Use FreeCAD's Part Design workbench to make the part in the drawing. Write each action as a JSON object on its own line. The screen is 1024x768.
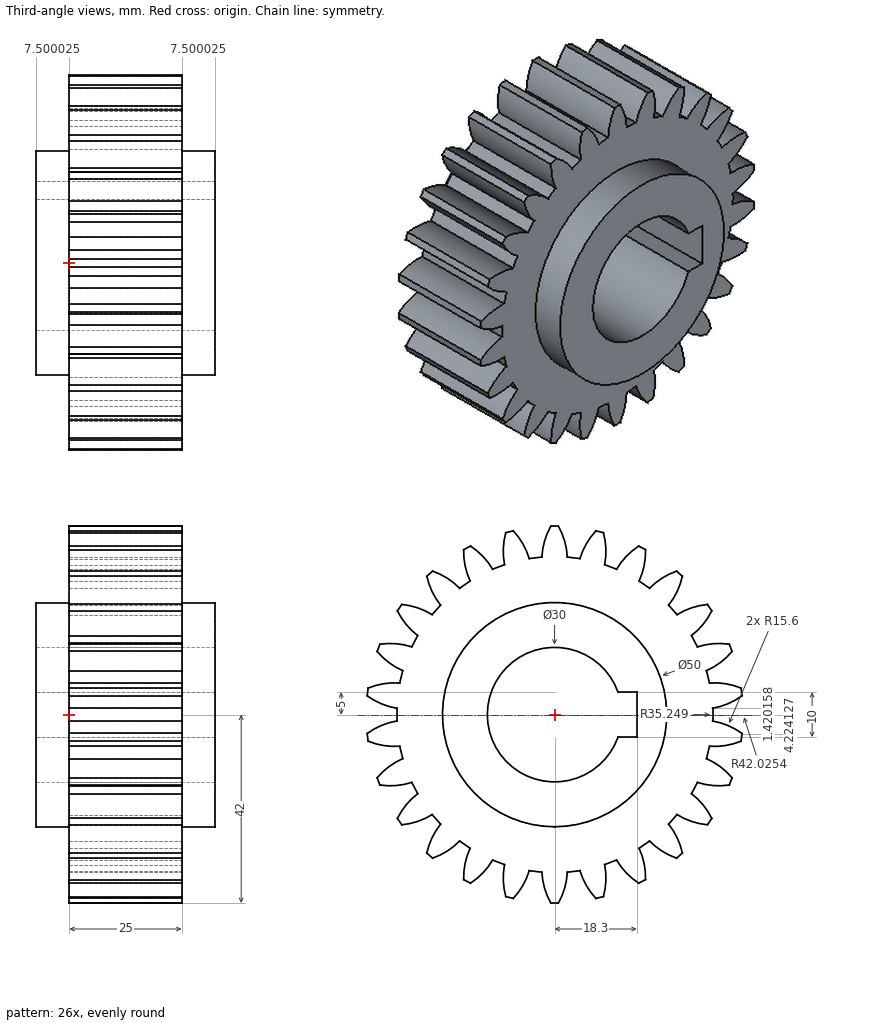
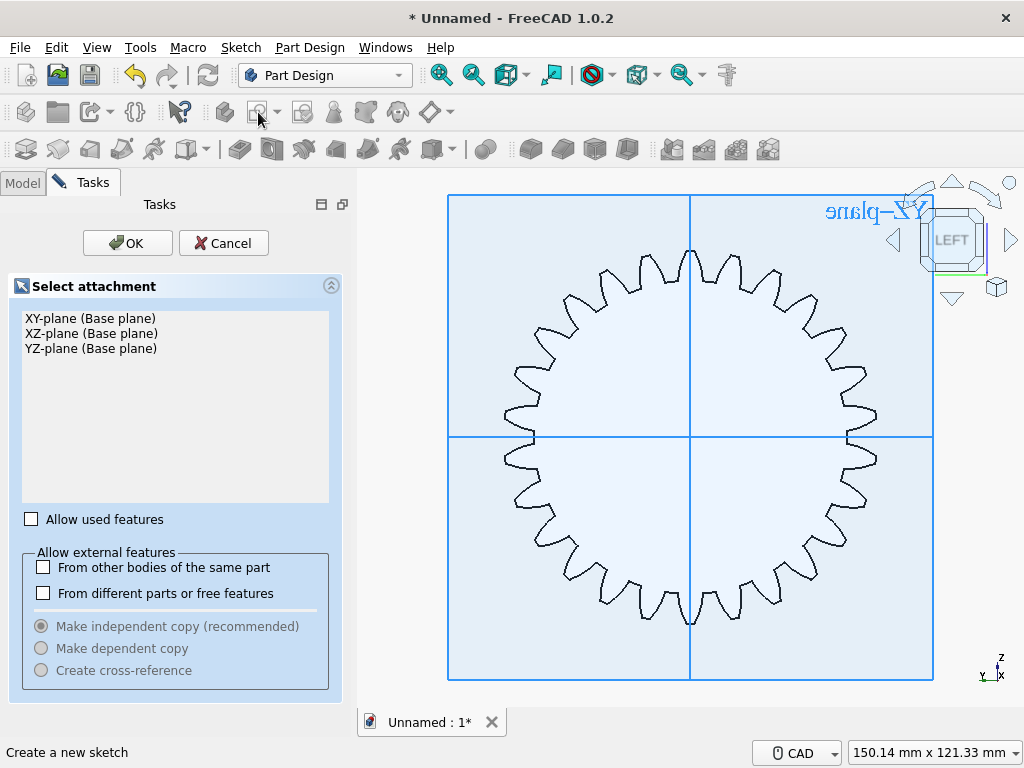
{"action": "left_click", "coordinate": [82, 348]}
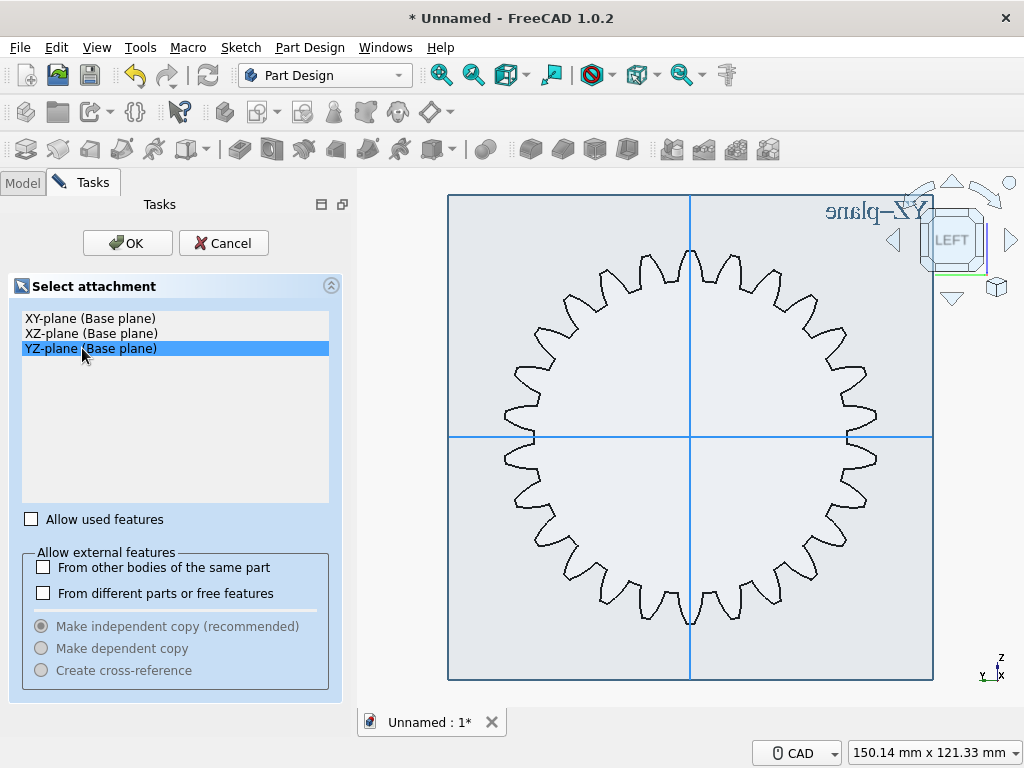
{"action": "left_click", "coordinate": [128, 243]}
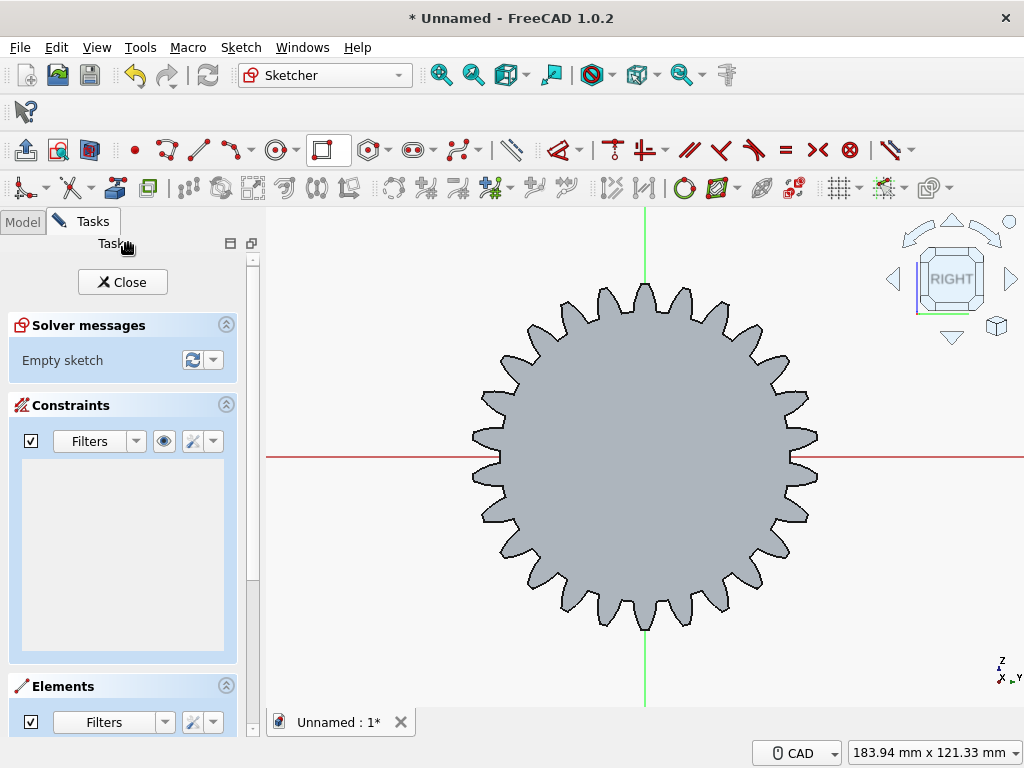
{"action": "left_click", "coordinate": [90, 150]}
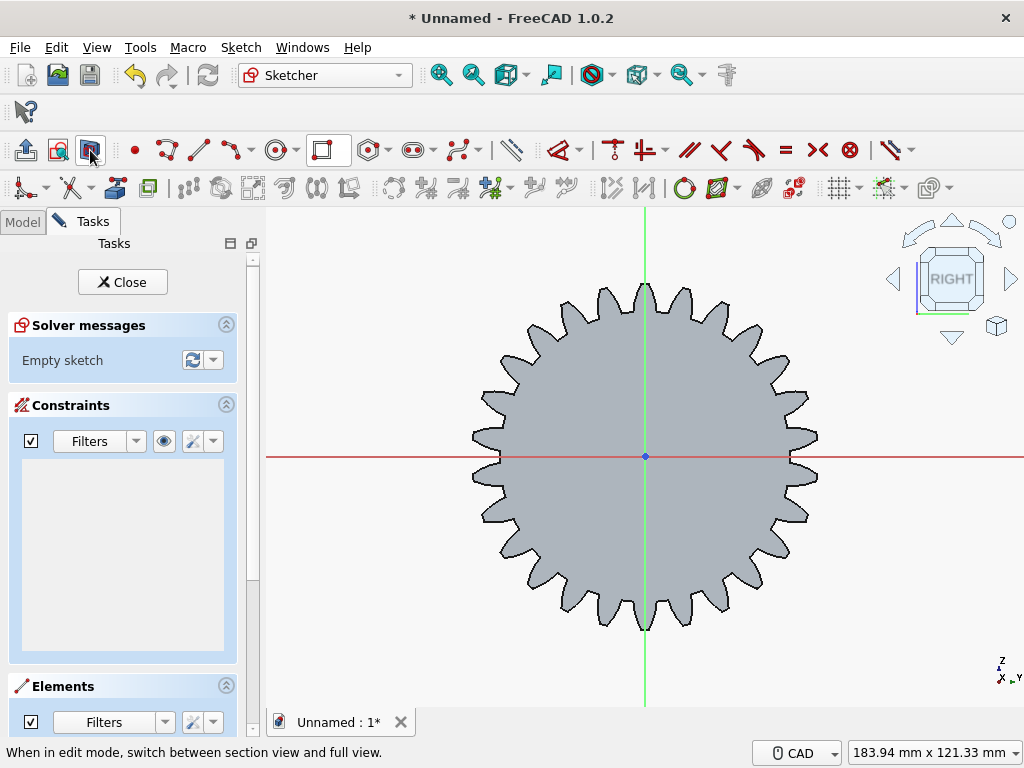
{"action": "scroll", "coordinate": [784, 457], "scroll_direction": "up", "scroll_amount": 2}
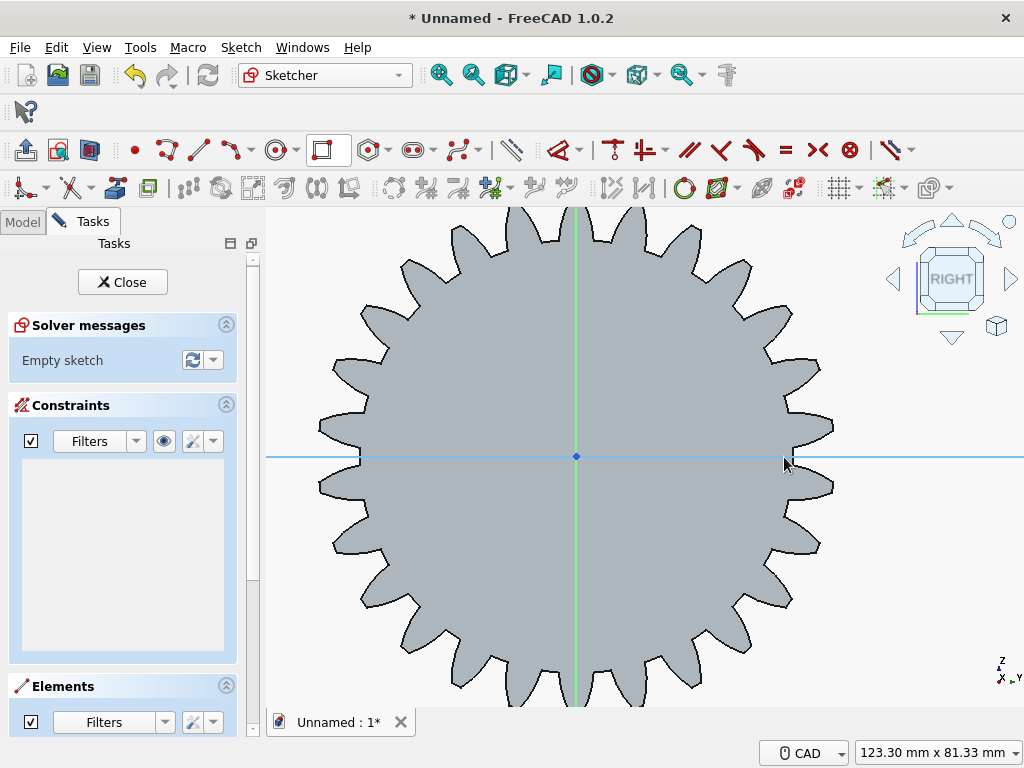
{"action": "left_click", "coordinate": [276, 150]}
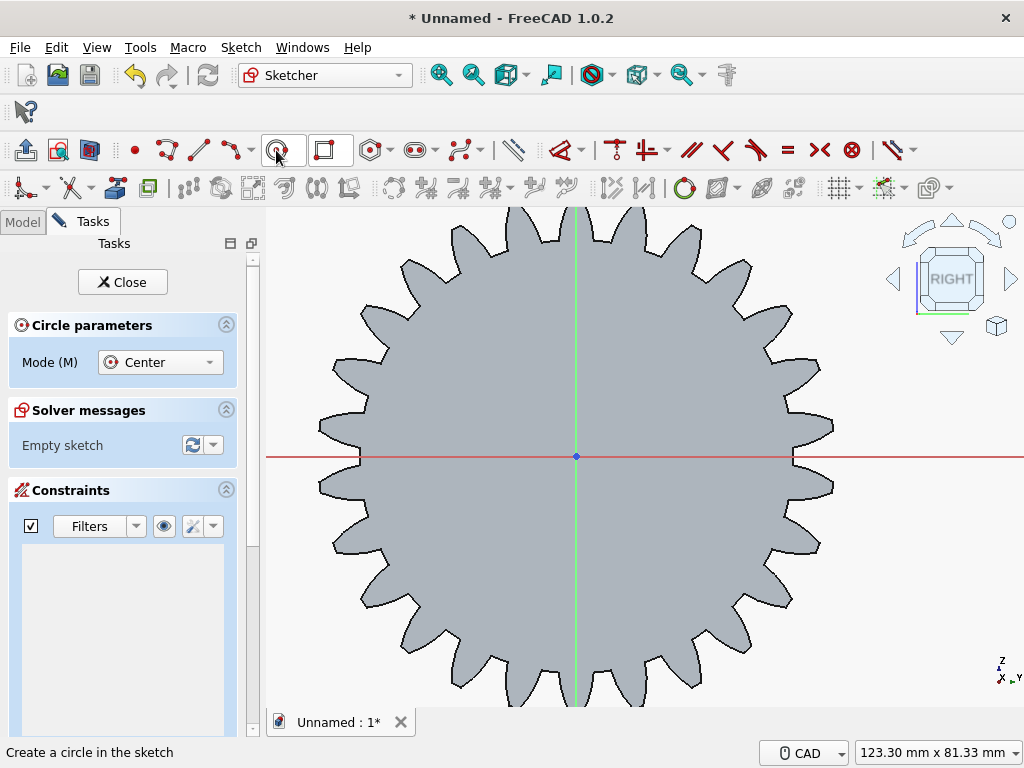
{"action": "left_click", "coordinate": [576, 457]}
{"action": "mouse_move", "coordinate": [685, 348]}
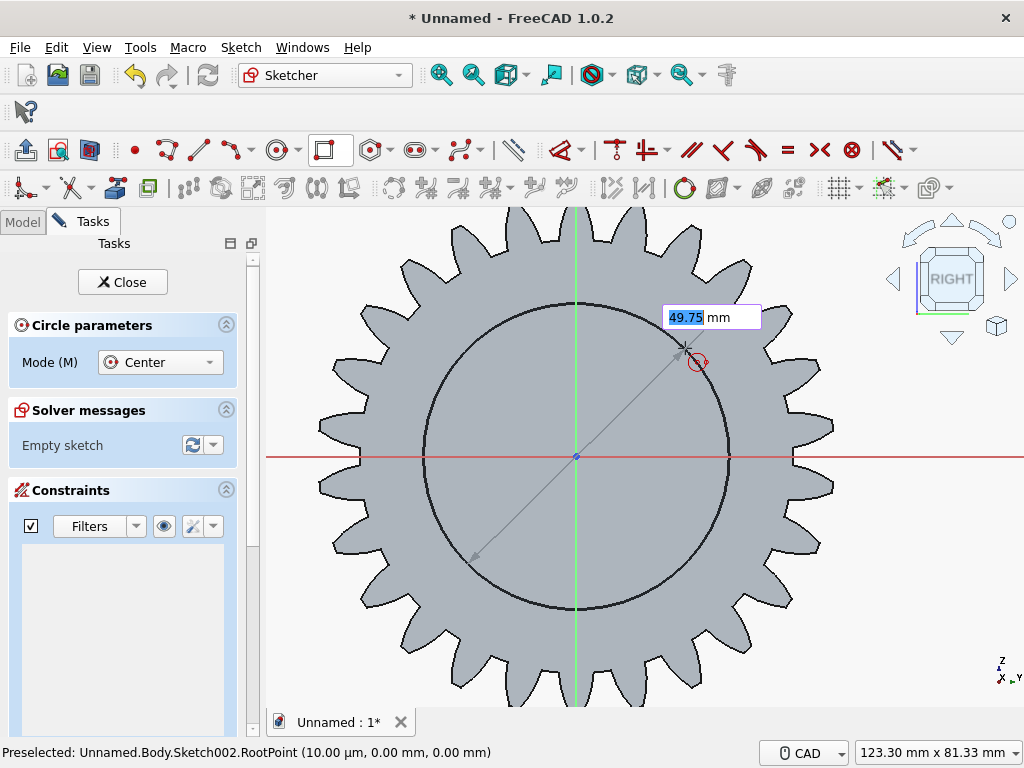
{"action": "type", "text": "50"}
{"action": "key", "text": "Return"}
{"action": "key", "text": "Escape"}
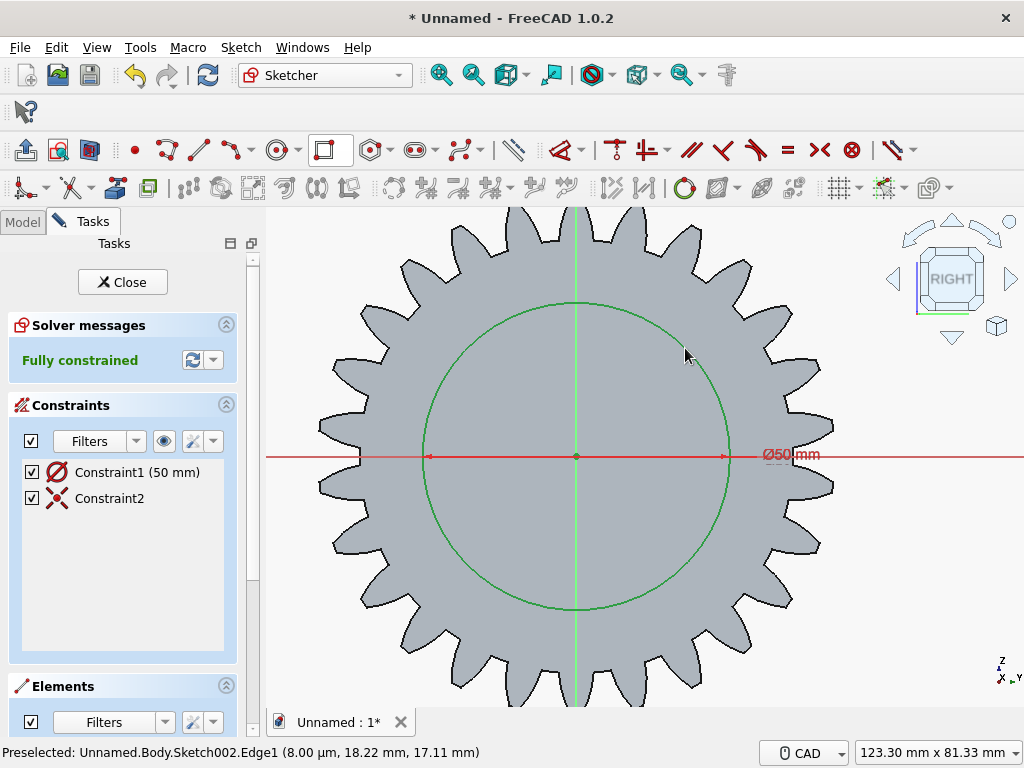
{"action": "left_click", "coordinate": [123, 282]}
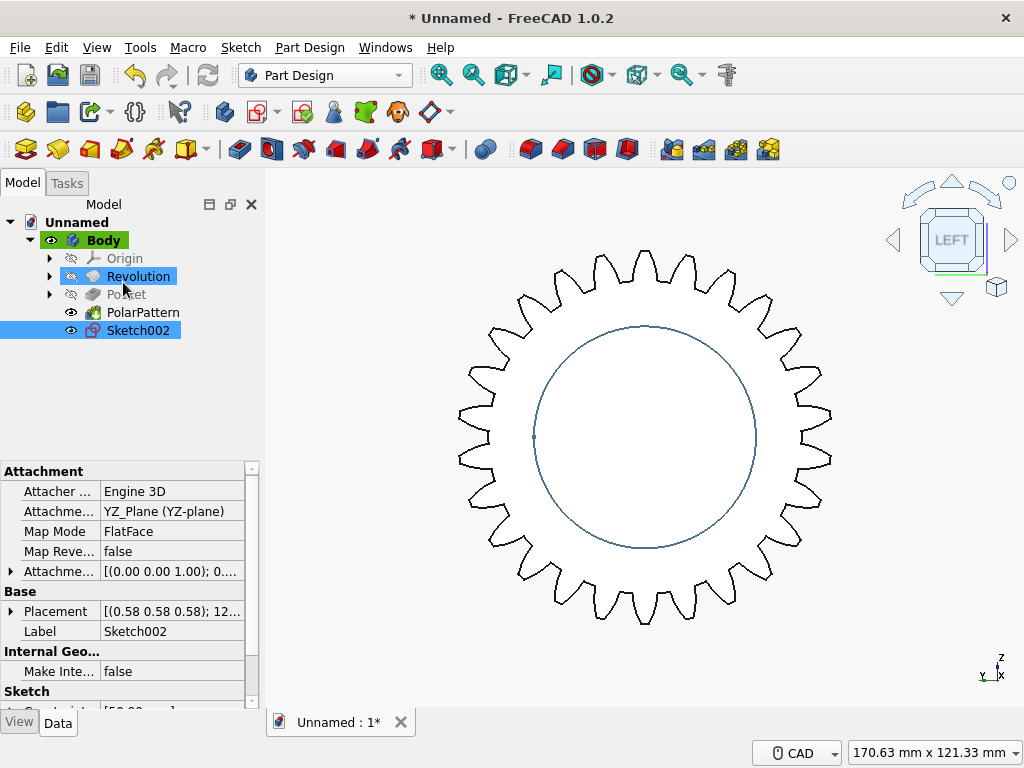
{"action": "left_click", "coordinate": [26, 150]}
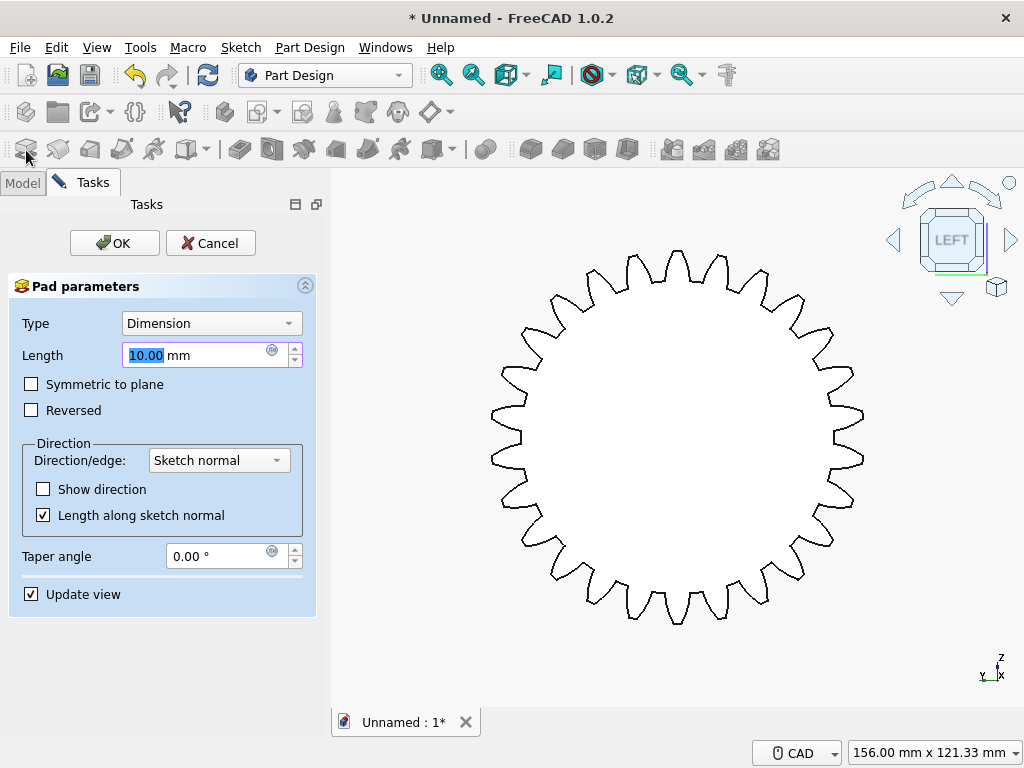
{"action": "type", "text": "7.500025"}
{"action": "key", "text": "Tab"}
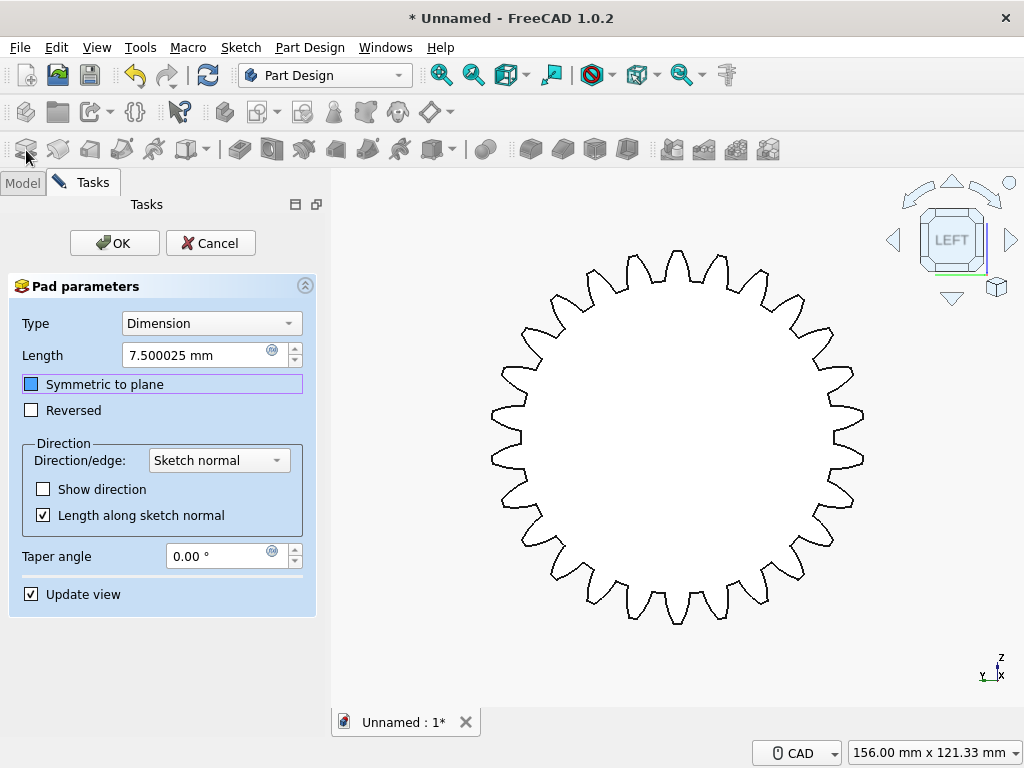
{"action": "left_click", "coordinate": [30, 410]}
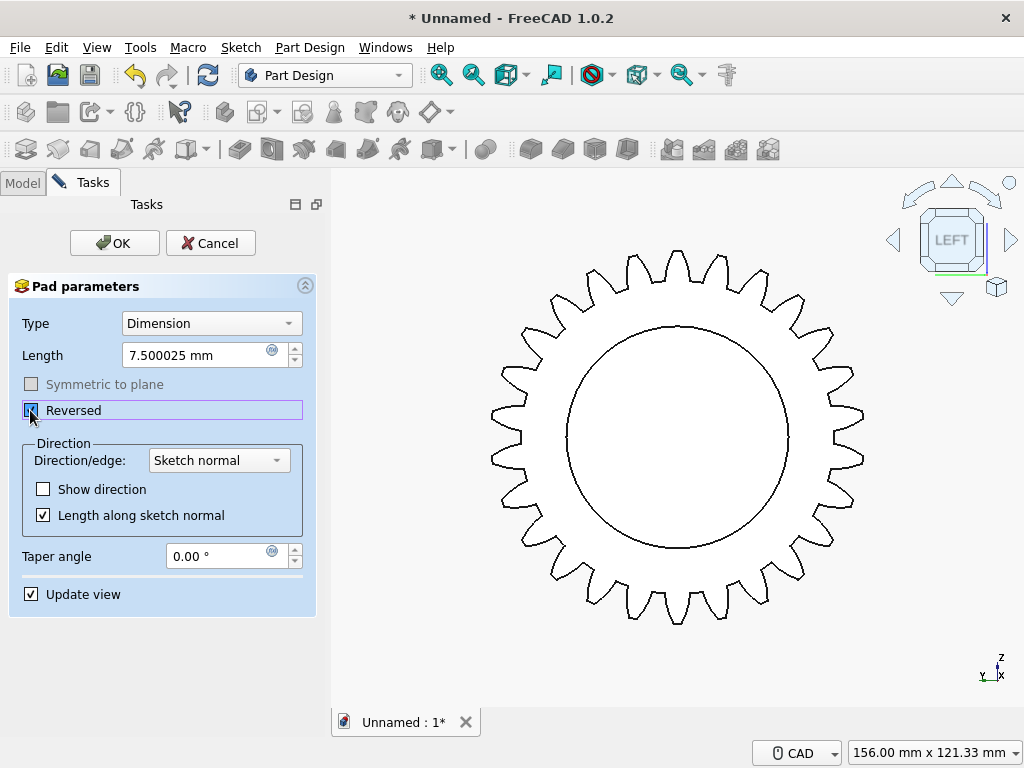
{"action": "left_click", "coordinate": [115, 243]}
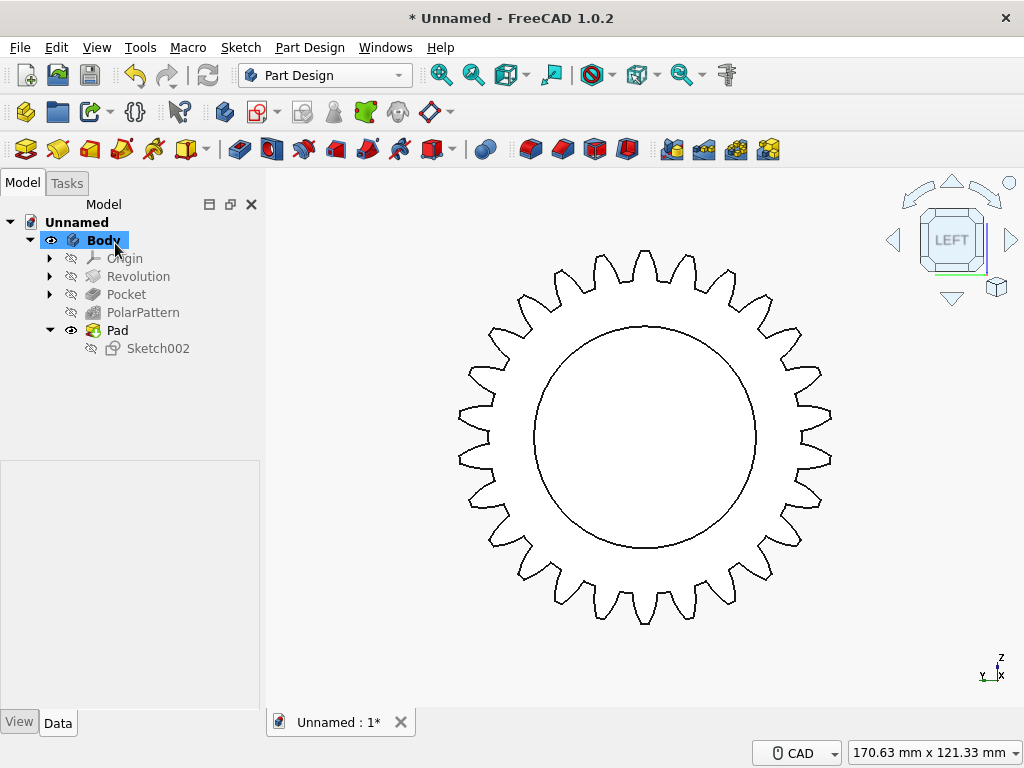
{"action": "left_click", "coordinate": [50, 258]}